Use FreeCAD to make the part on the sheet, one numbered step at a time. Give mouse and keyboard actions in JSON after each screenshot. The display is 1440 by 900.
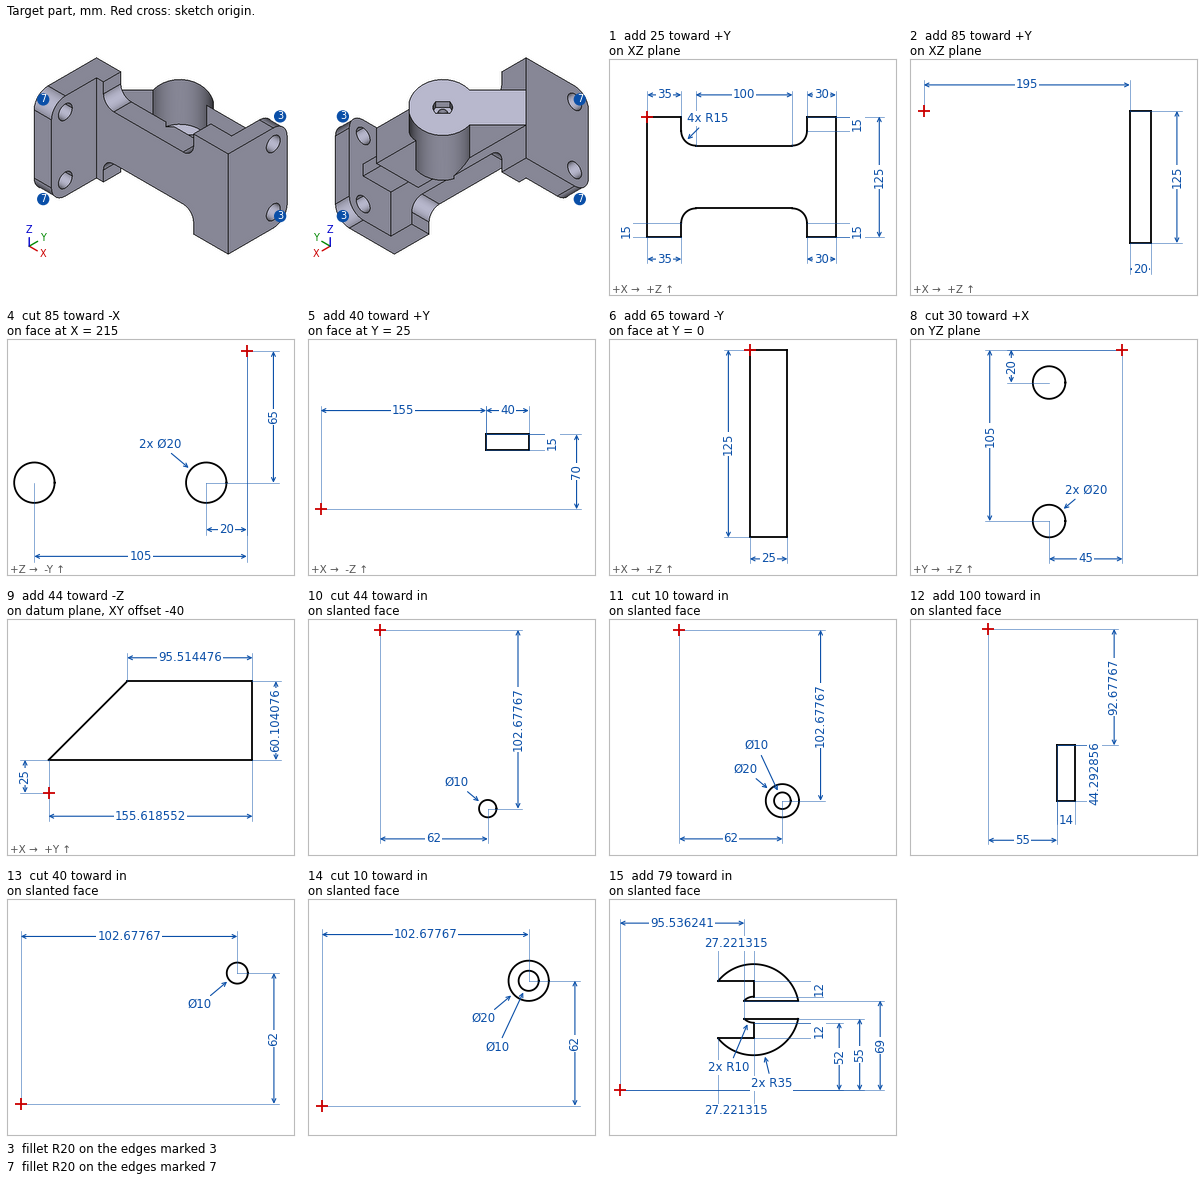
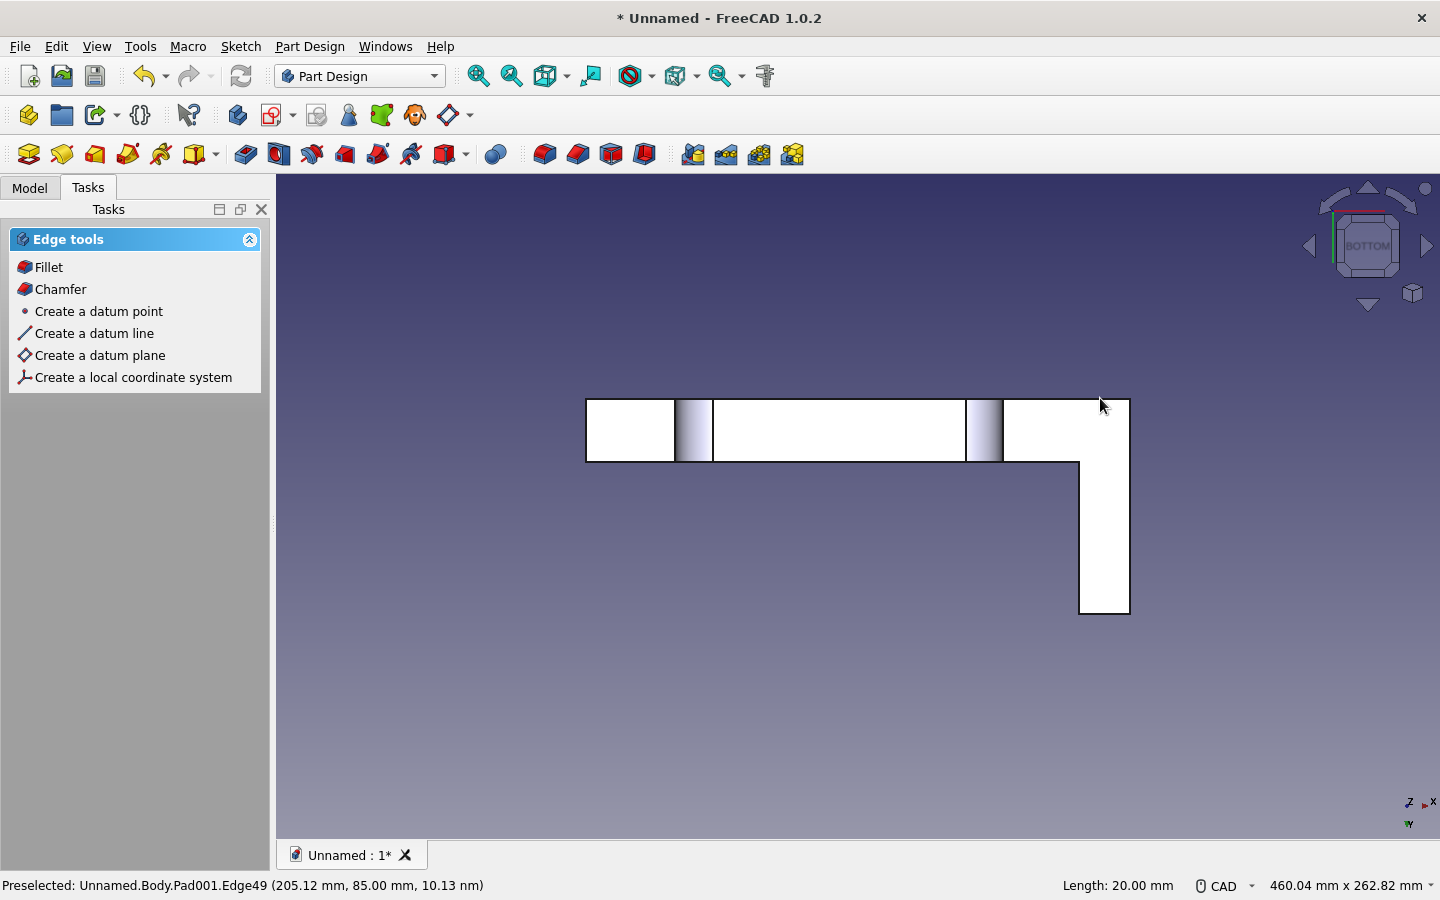
{"action": "key", "text": "4"}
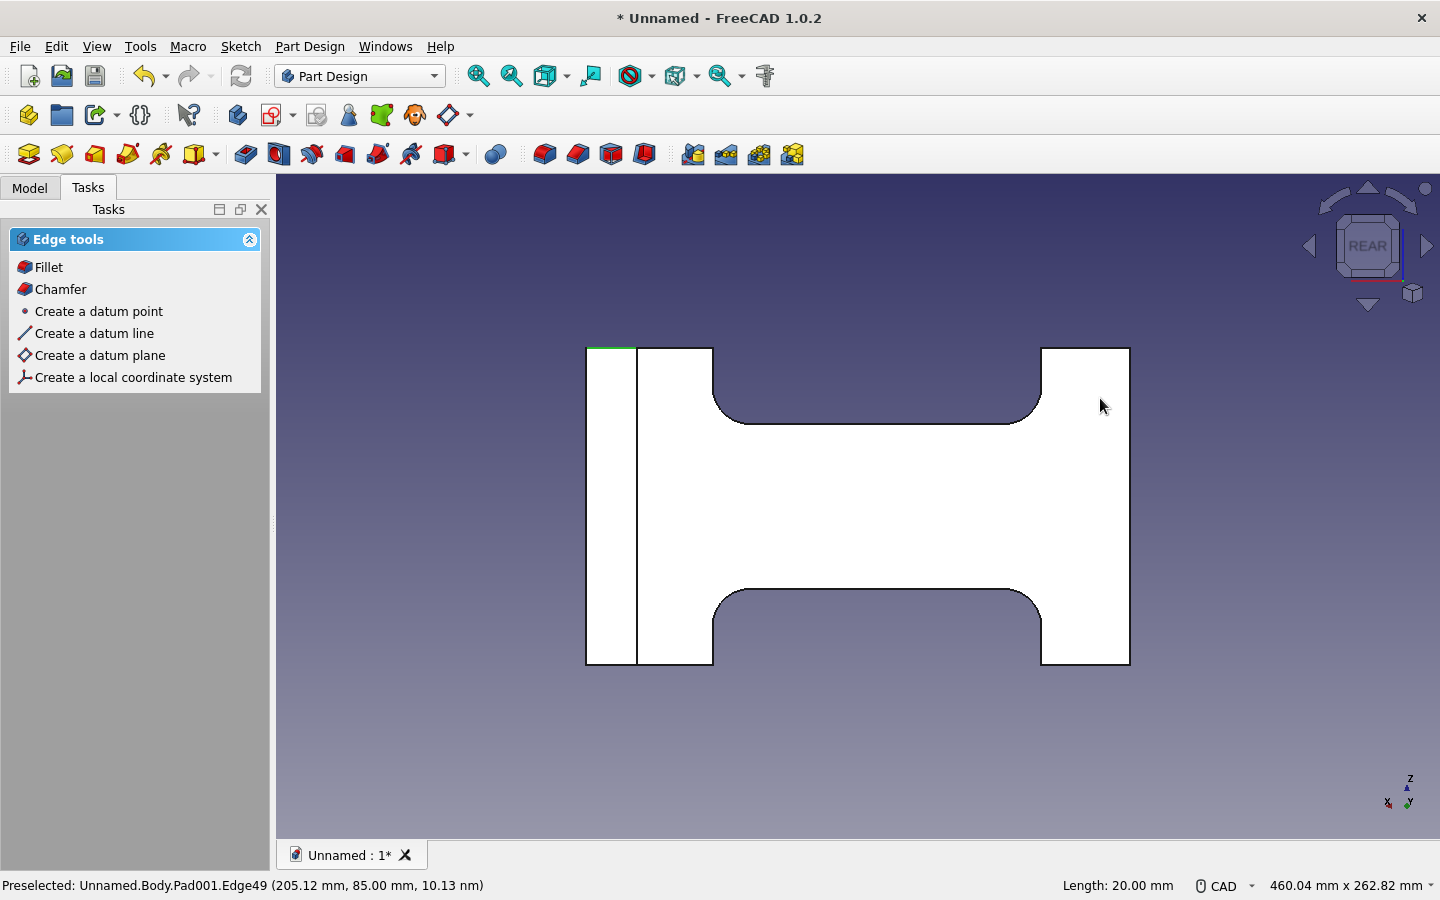
{"action": "left_click", "coordinate": [611, 664], "text": "ctrl"}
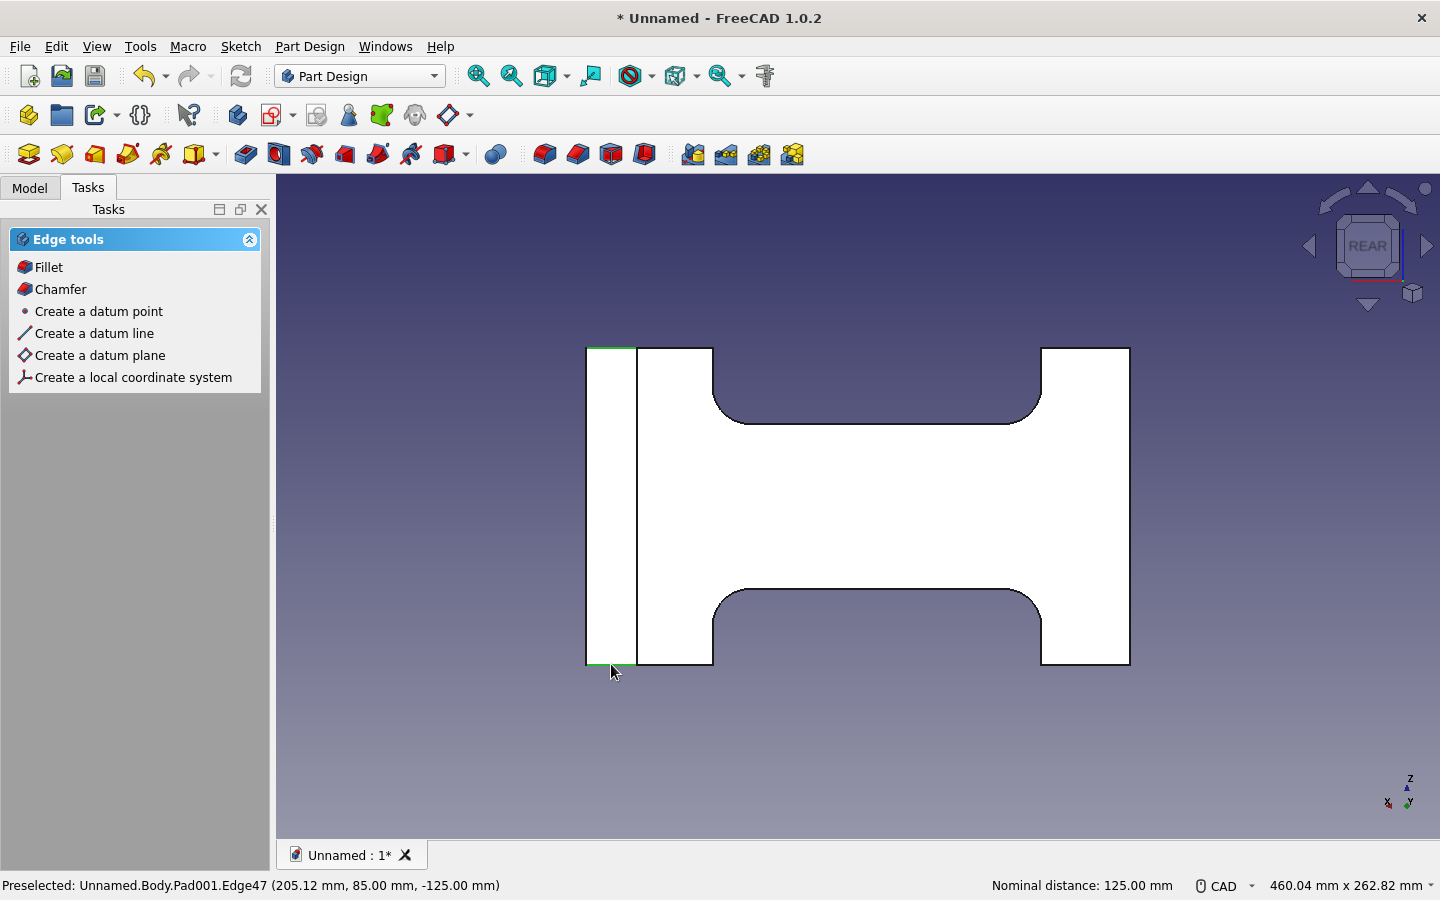
{"action": "left_click", "coordinate": [545, 154]}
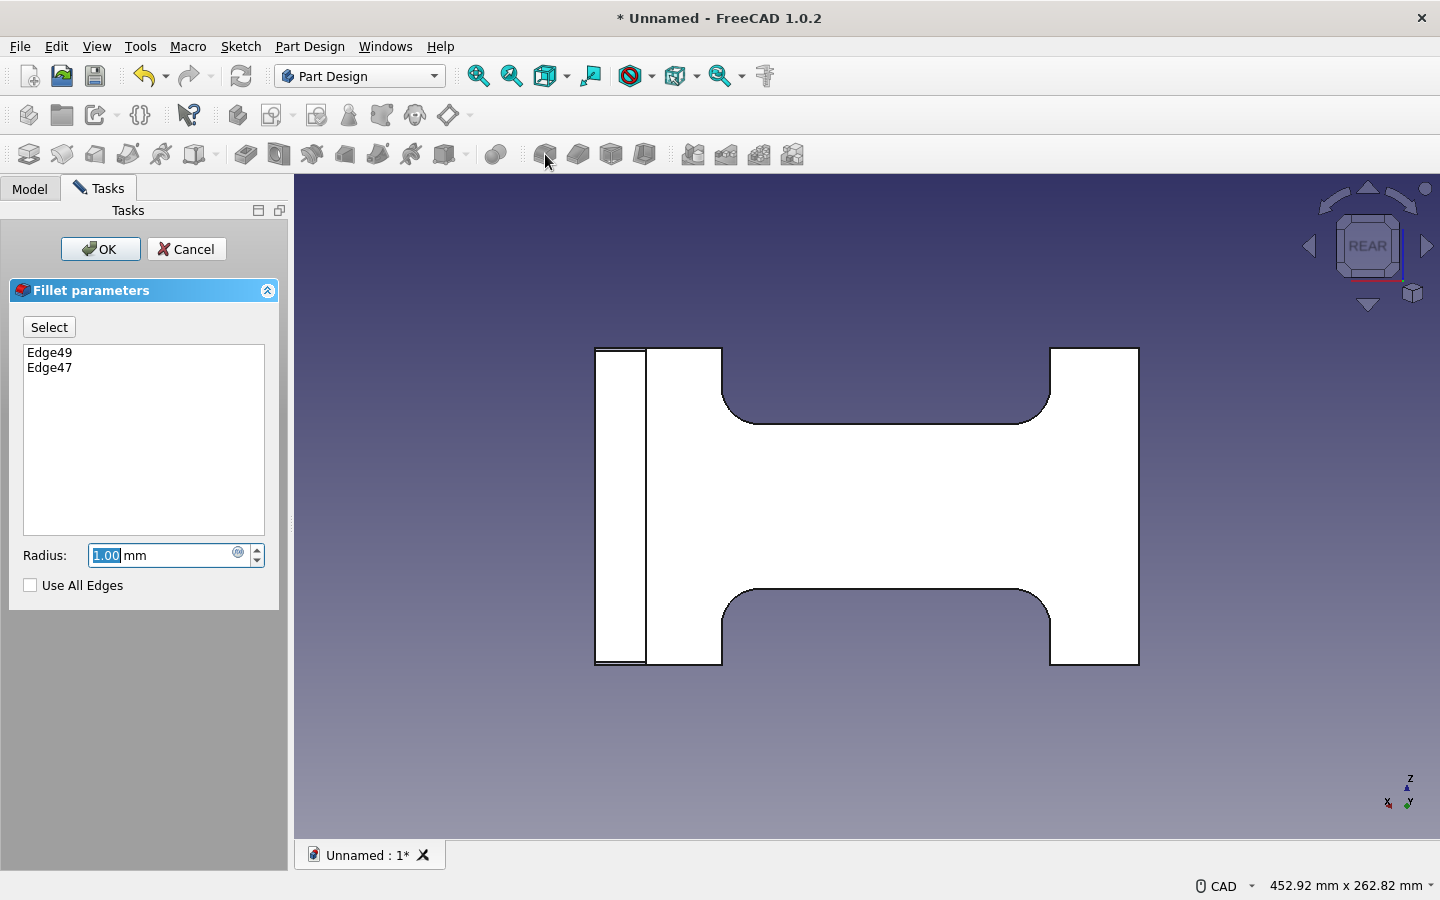
{"action": "type", "text": "20"}
{"action": "key", "text": "Tab"}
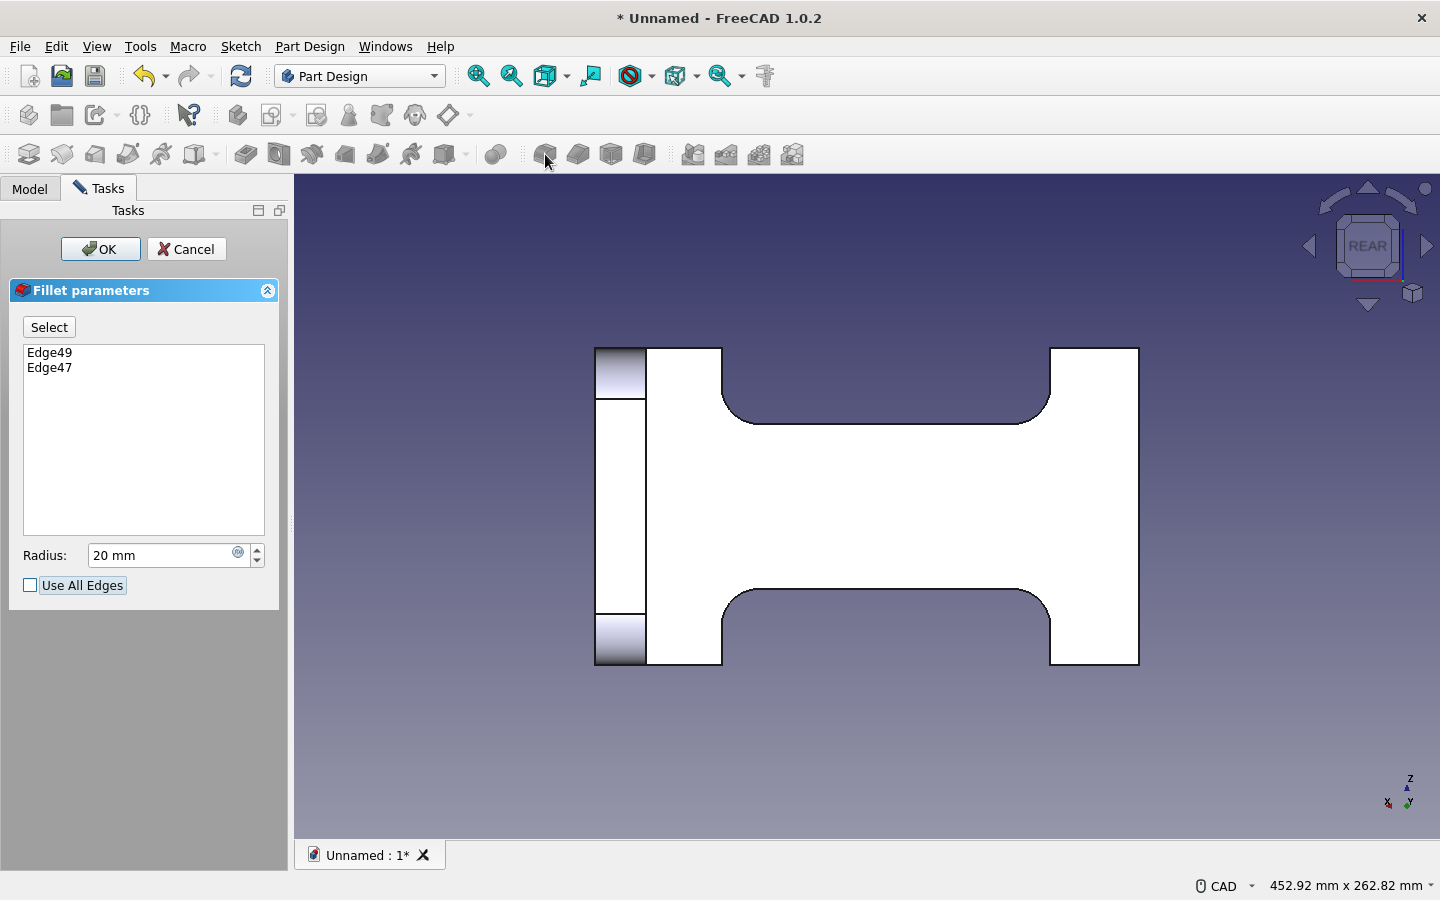
{"action": "left_click", "coordinate": [101, 249]}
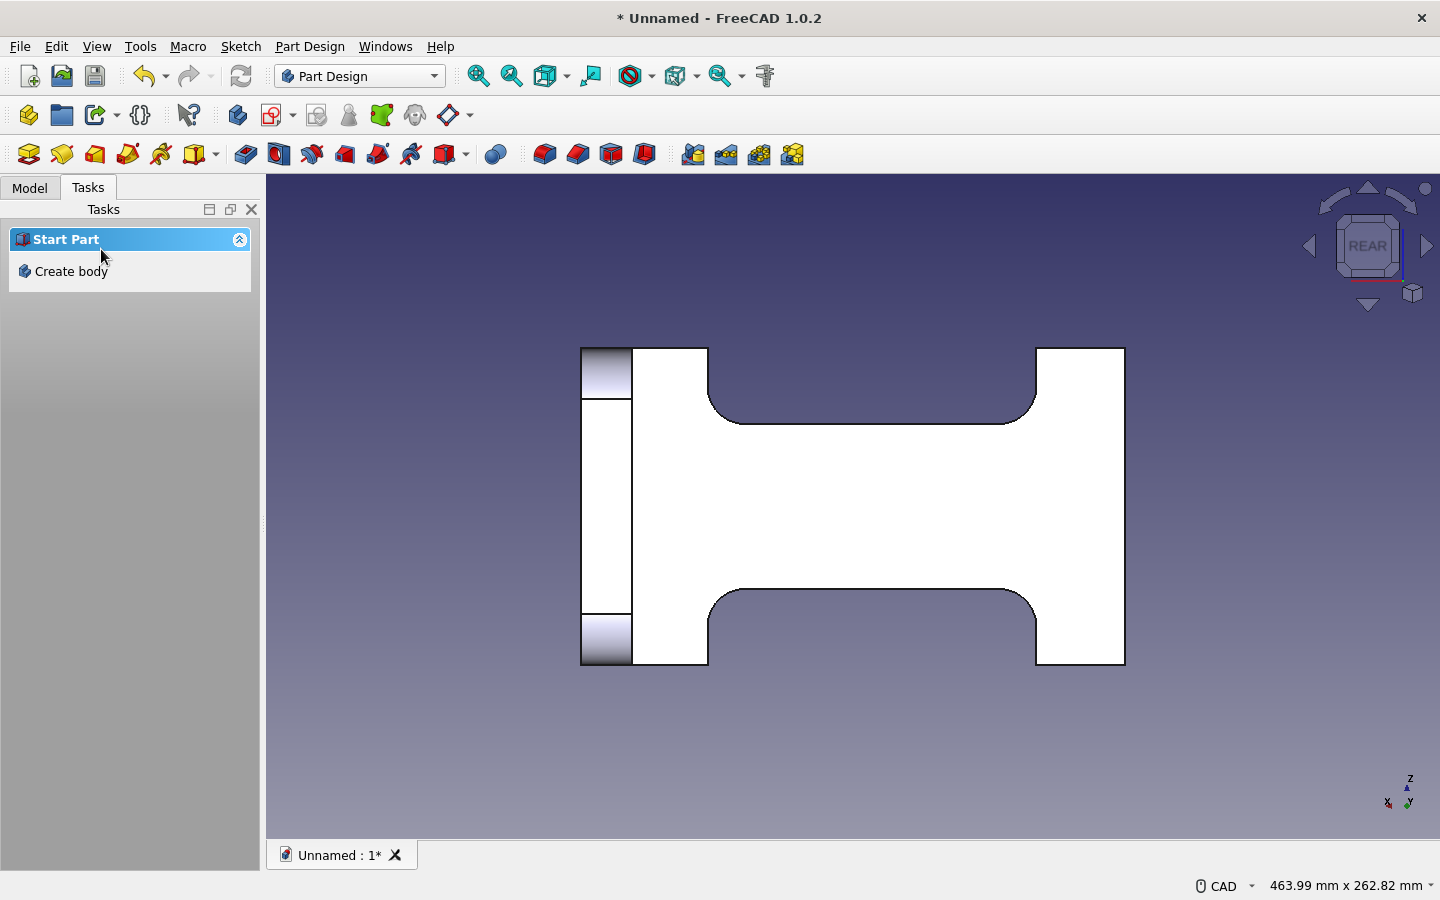
{"action": "key", "text": "0"}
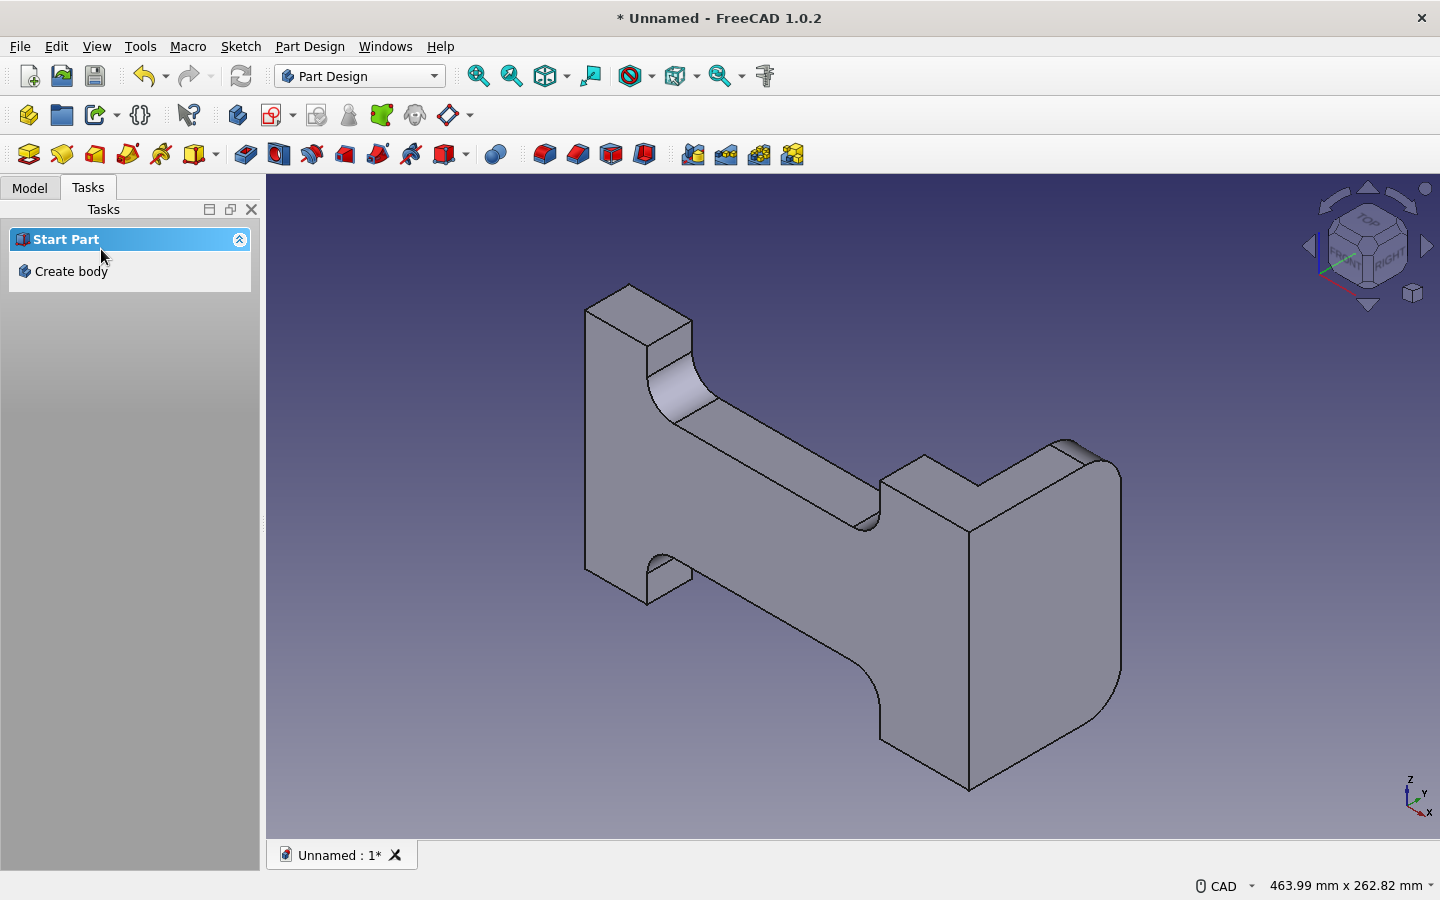
{"action": "left_click", "coordinate": [1045, 580]}